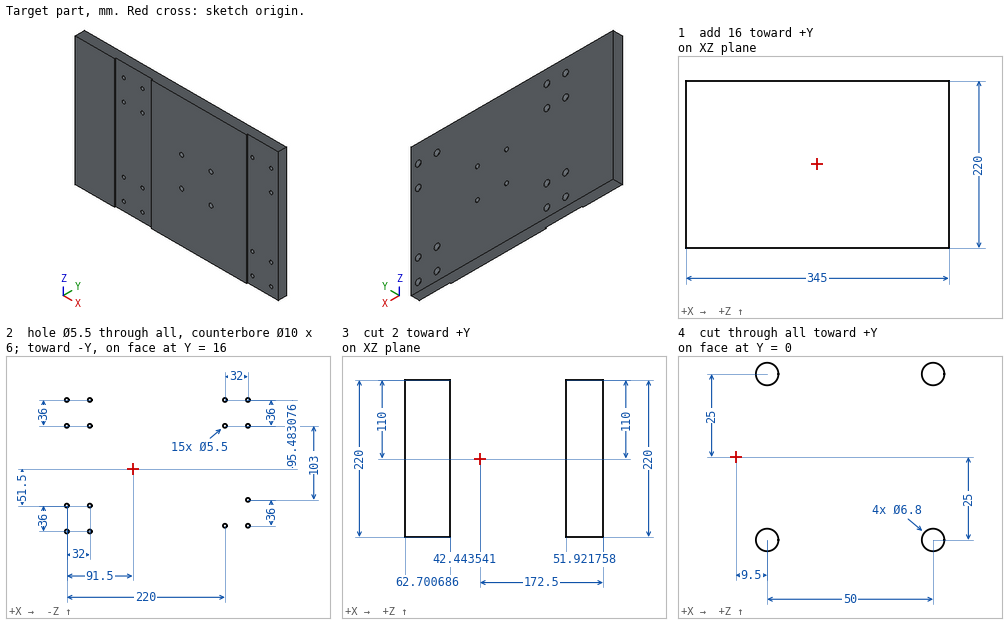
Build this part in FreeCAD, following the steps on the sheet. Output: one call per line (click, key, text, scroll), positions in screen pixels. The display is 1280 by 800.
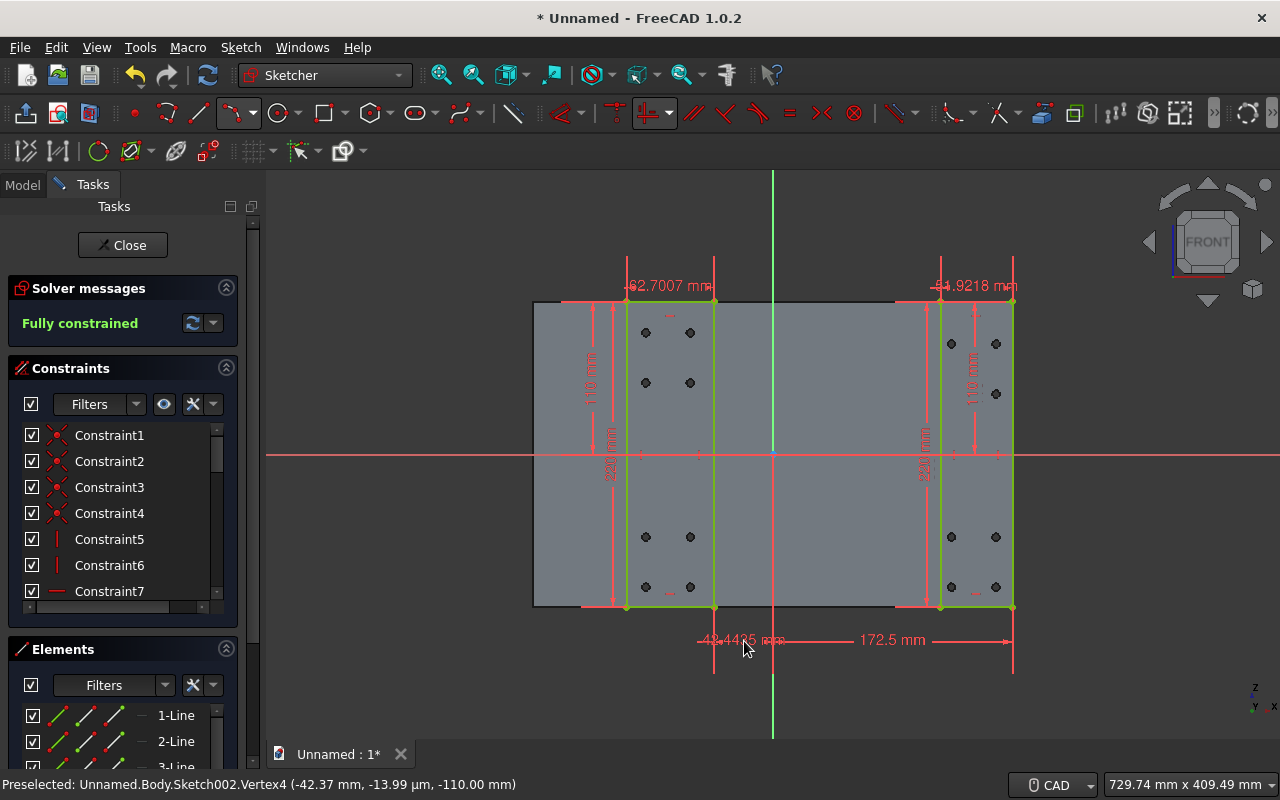
click(123, 245)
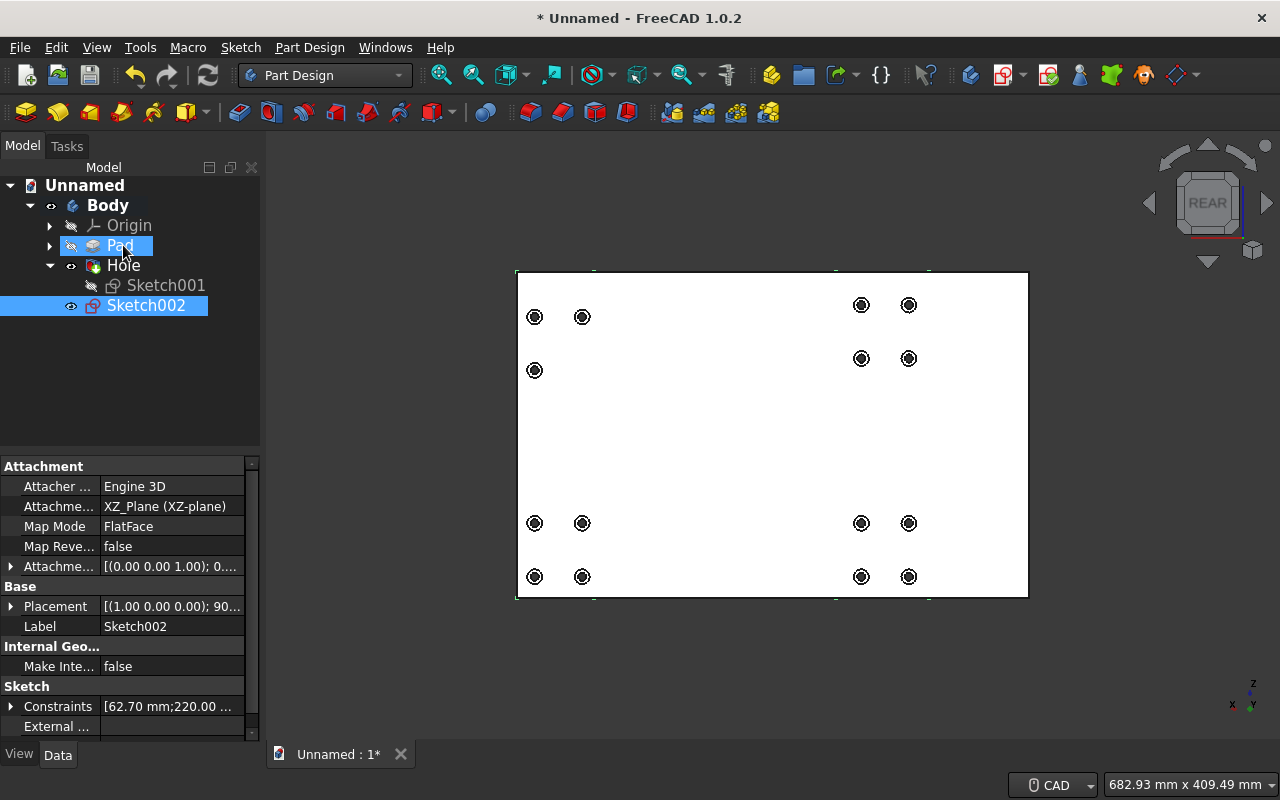
click(240, 112)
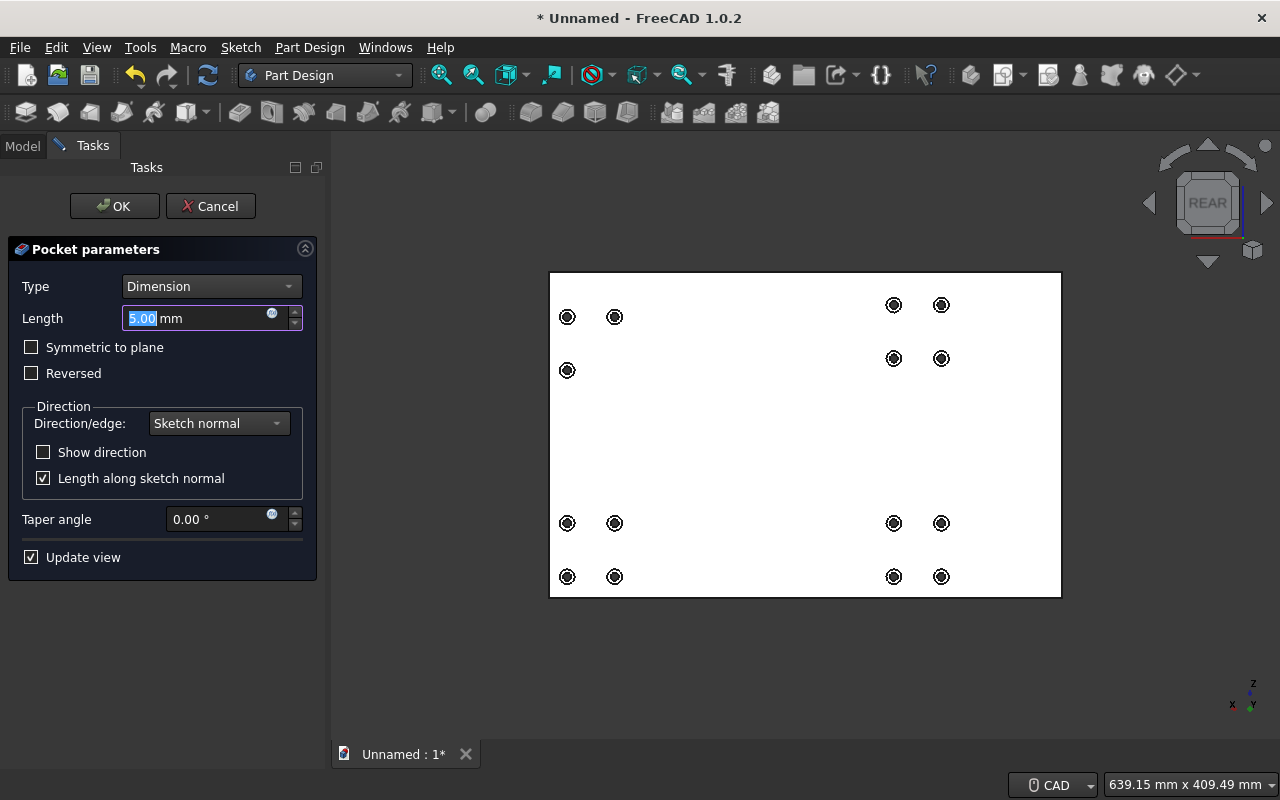
text(2)
key(Tab)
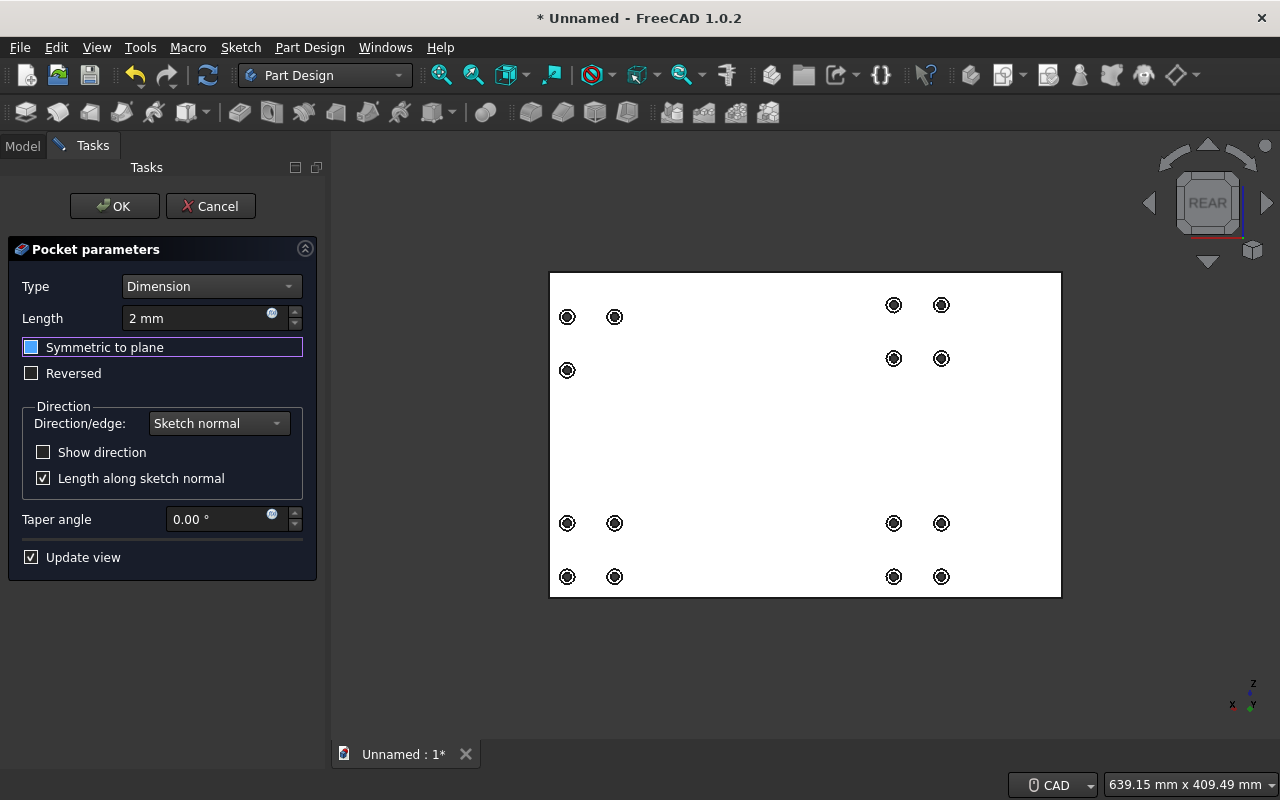
click(115, 206)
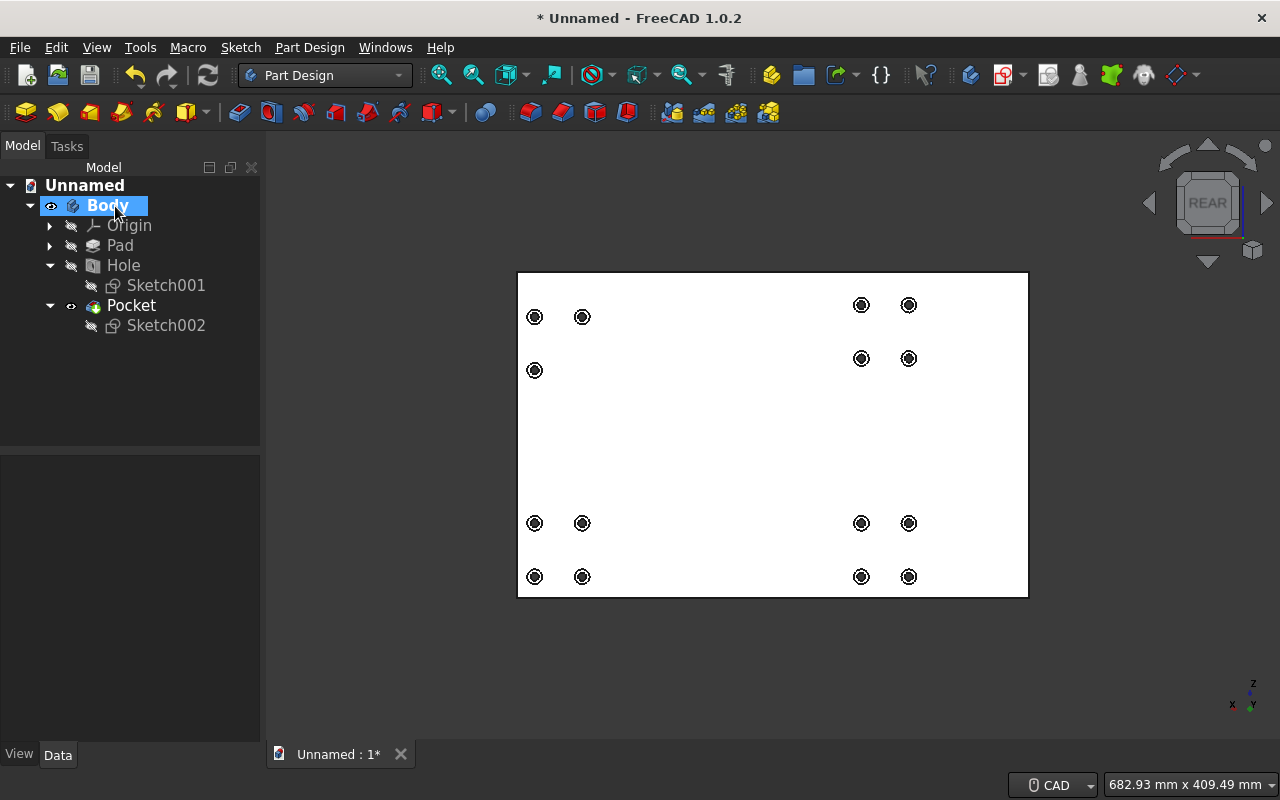
key(0)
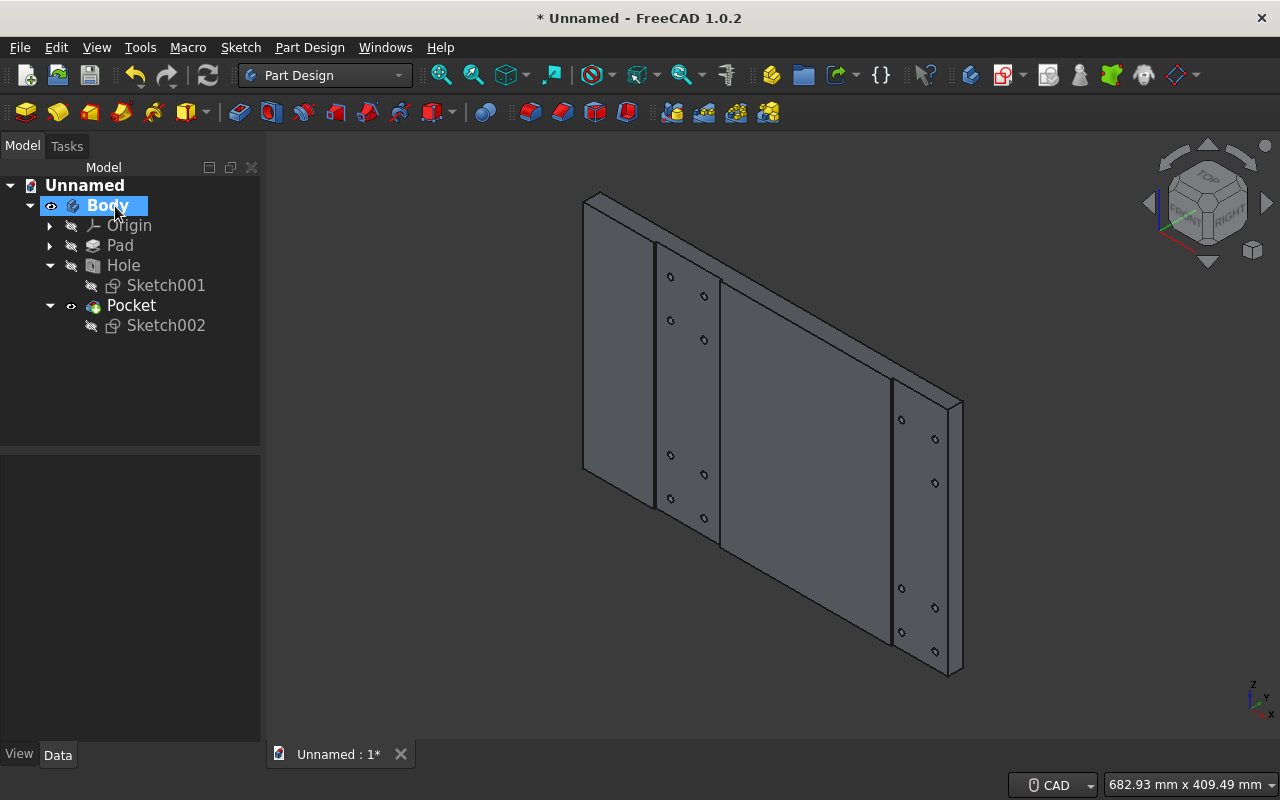
click(806, 463)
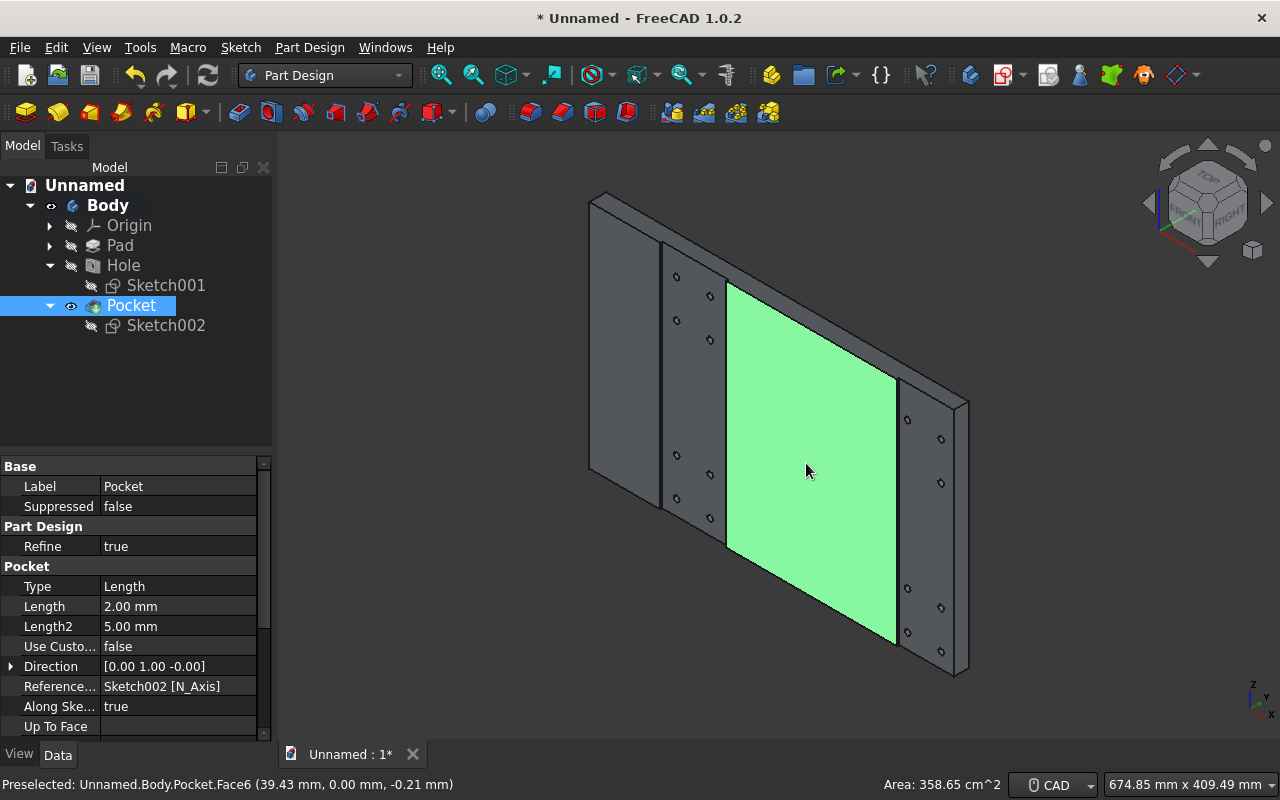
click(1004, 76)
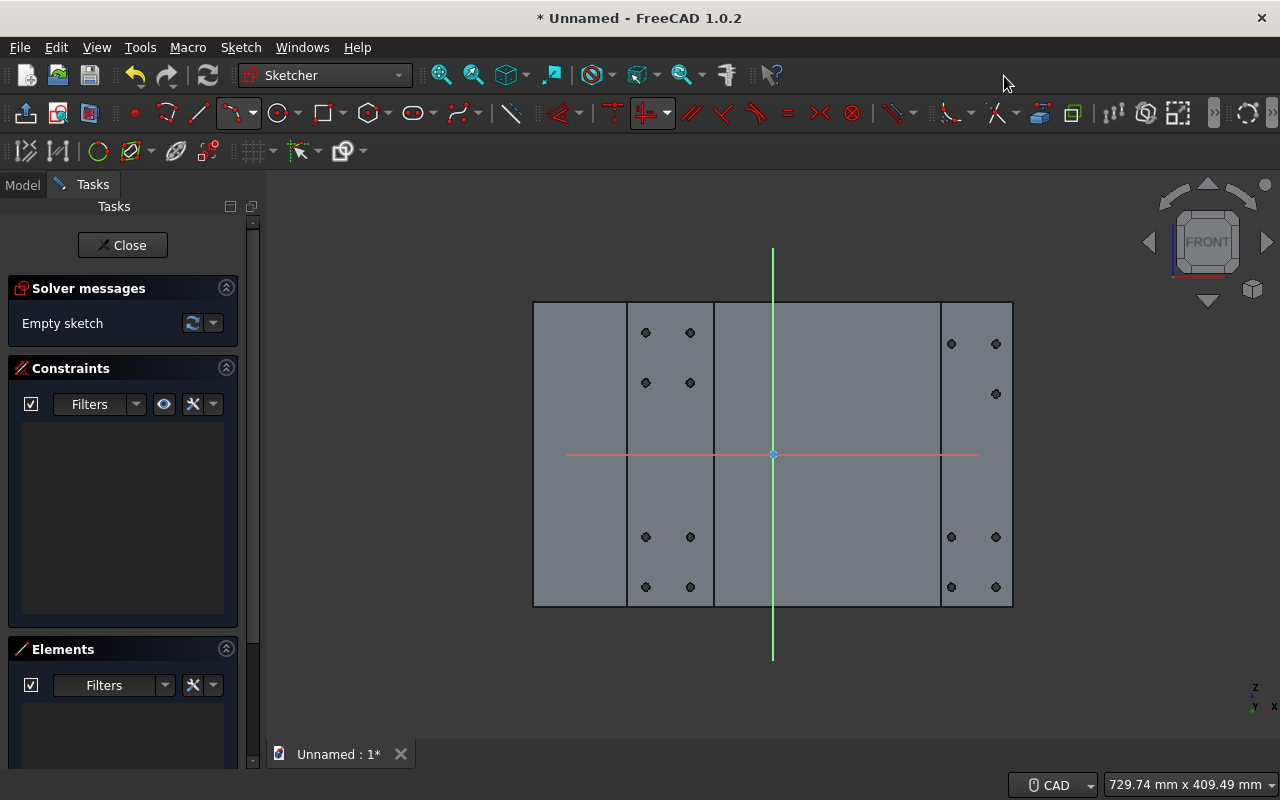
scroll(845, 455, up, 8)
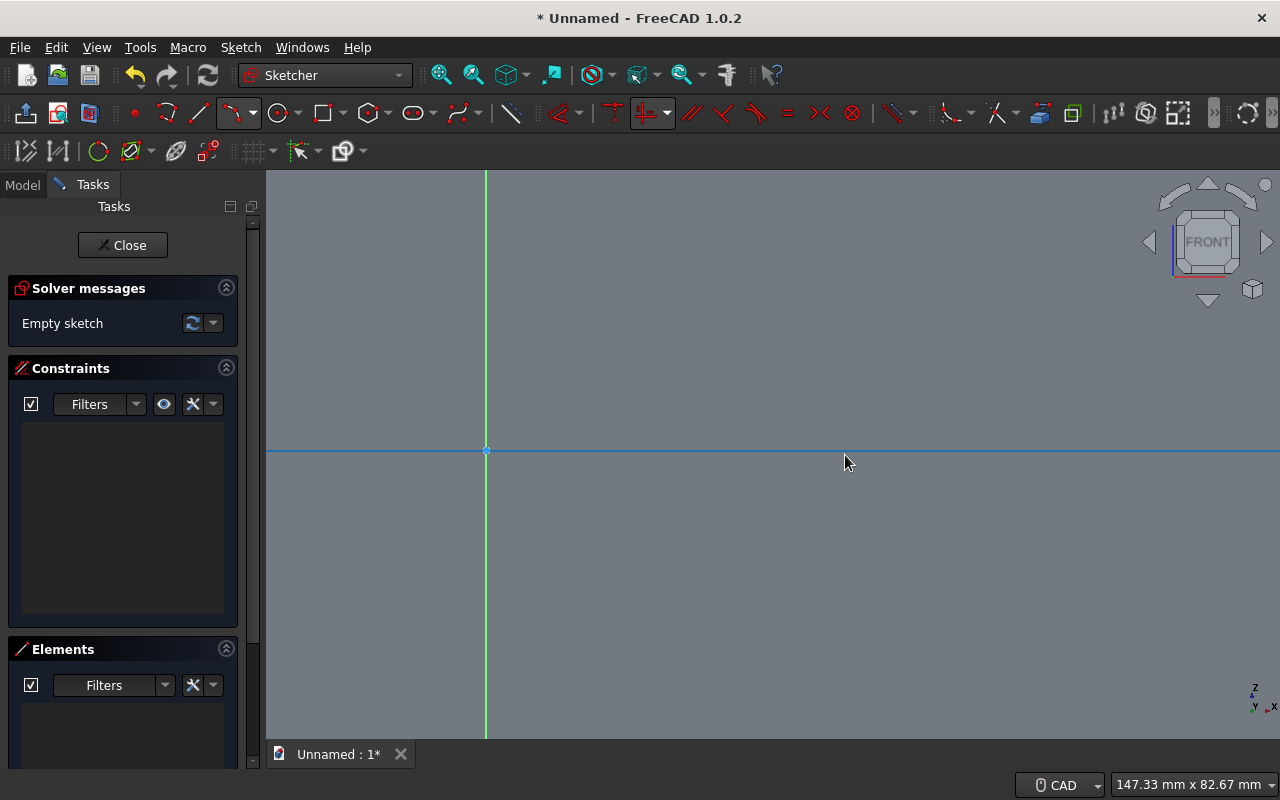
click(278, 114)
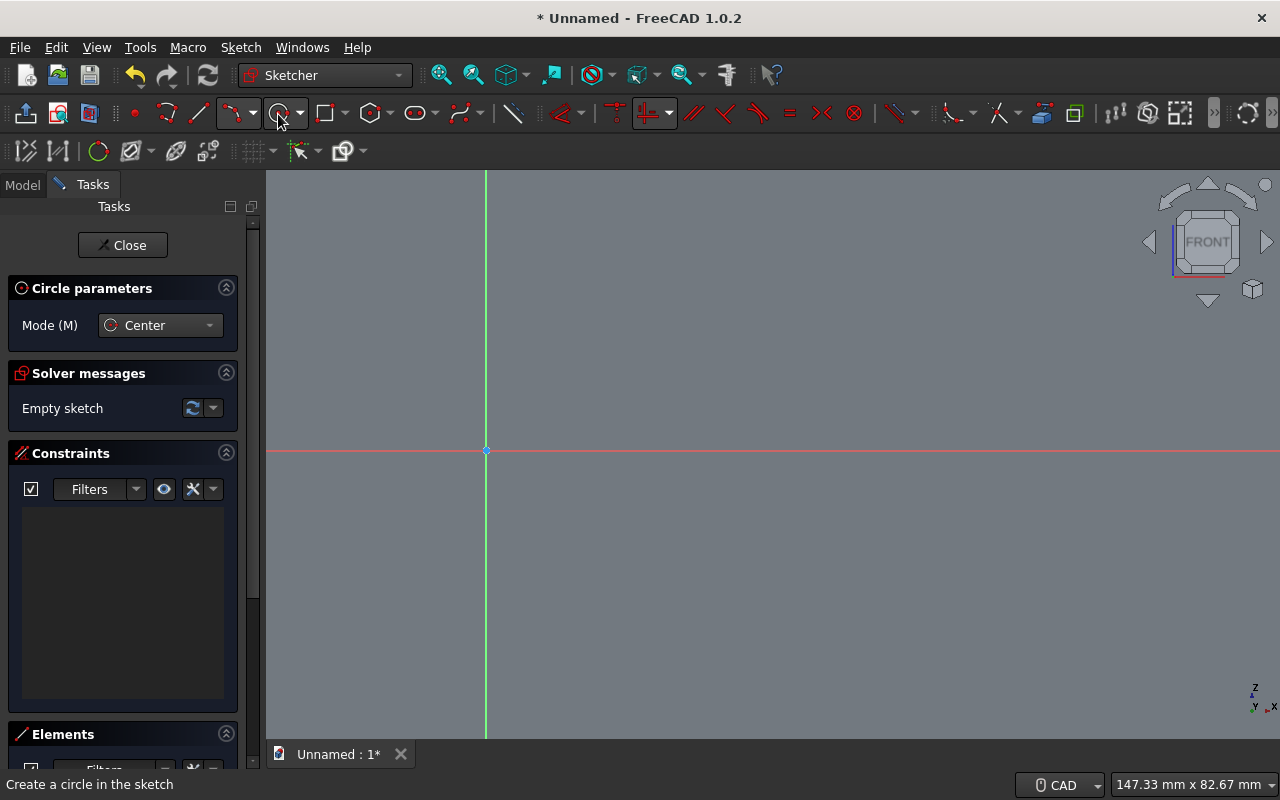
click(896, 623)
move(912, 606)